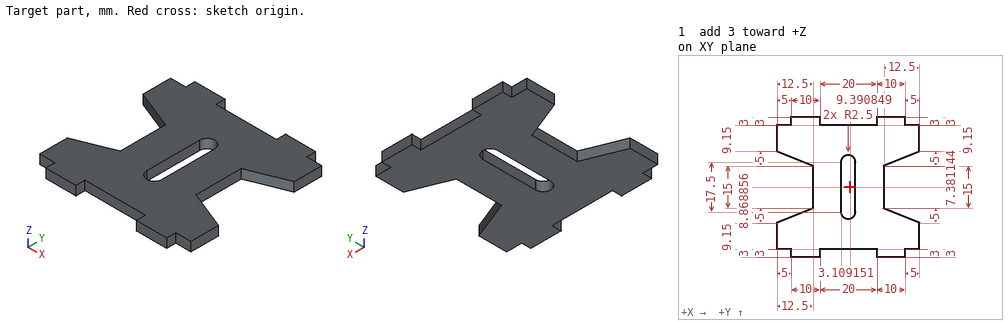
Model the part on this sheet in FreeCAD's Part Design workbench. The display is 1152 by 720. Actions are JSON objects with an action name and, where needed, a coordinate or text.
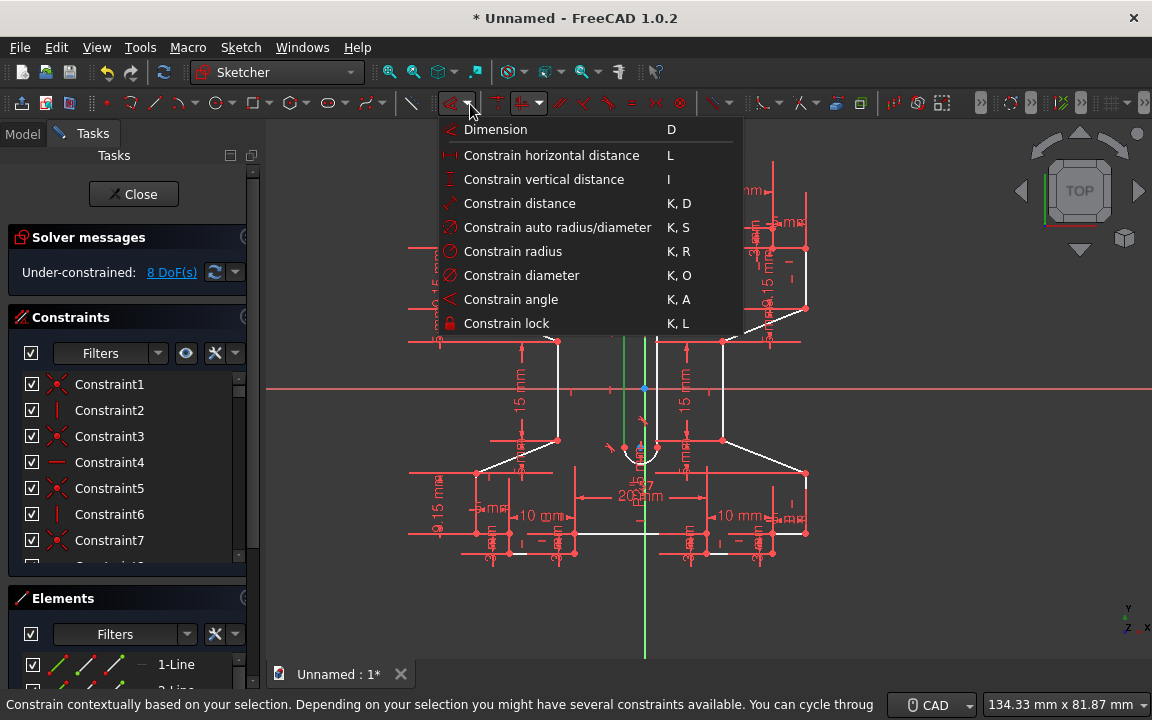
{"action": "left_click", "coordinate": [591, 179]}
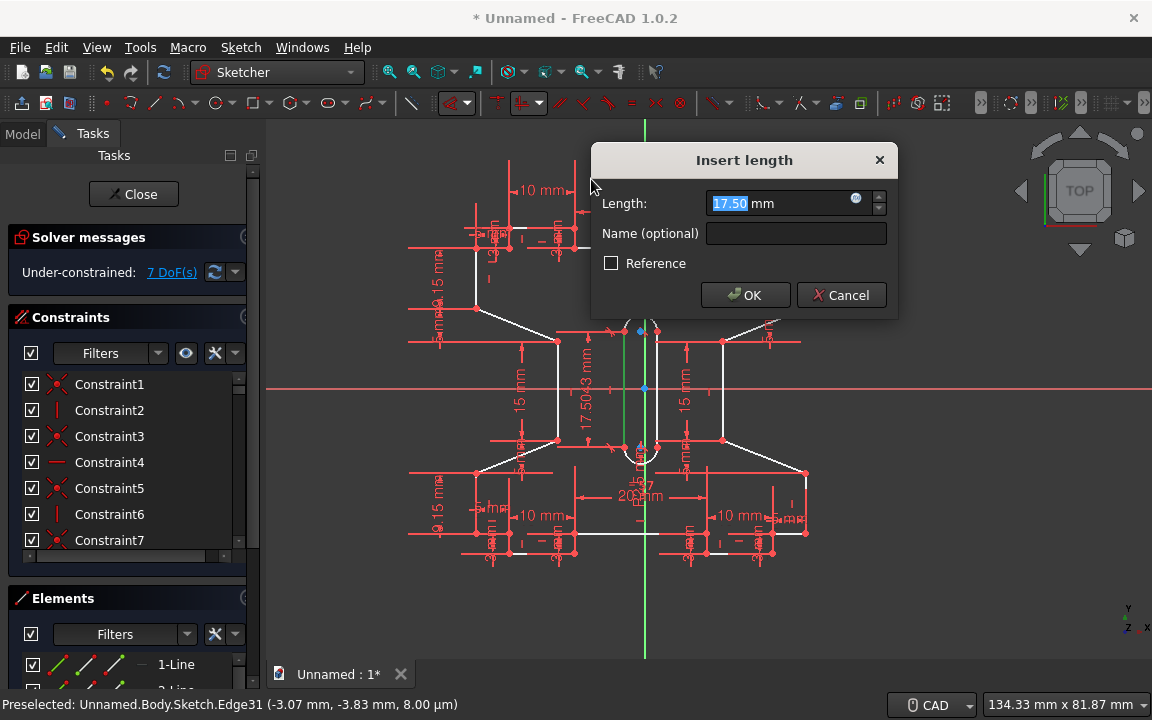
{"action": "type", "text": "17.5"}
{"action": "key", "text": "Return"}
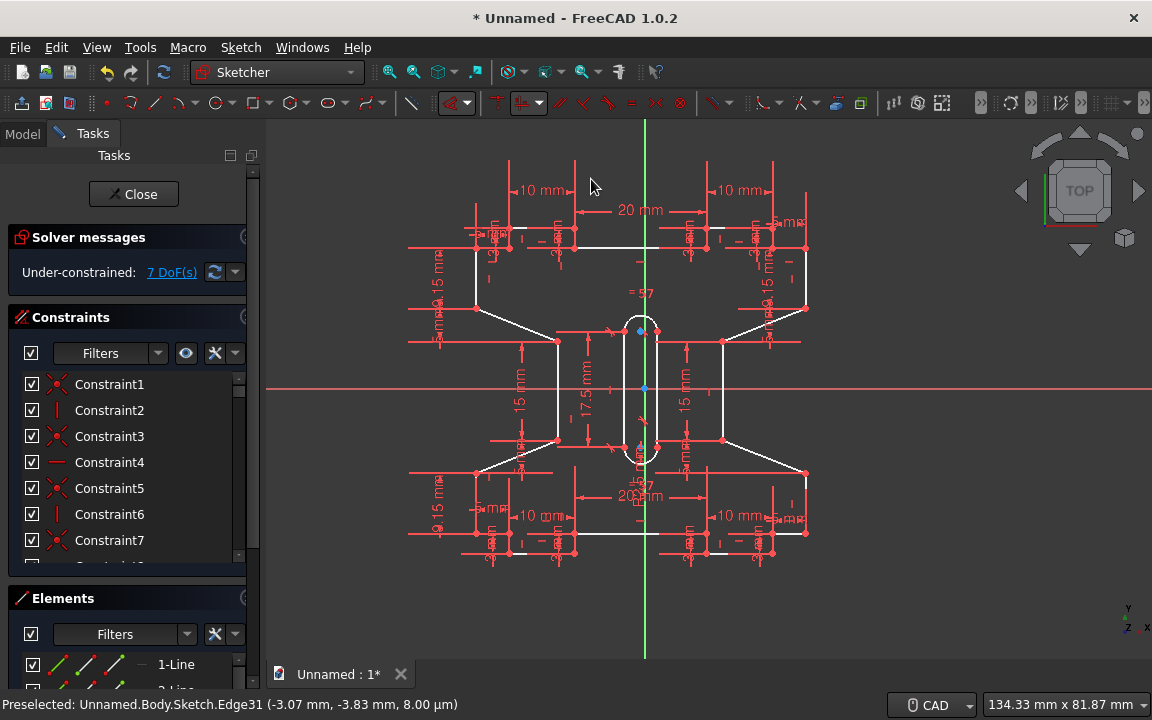
{"action": "left_click", "coordinate": [748, 332]}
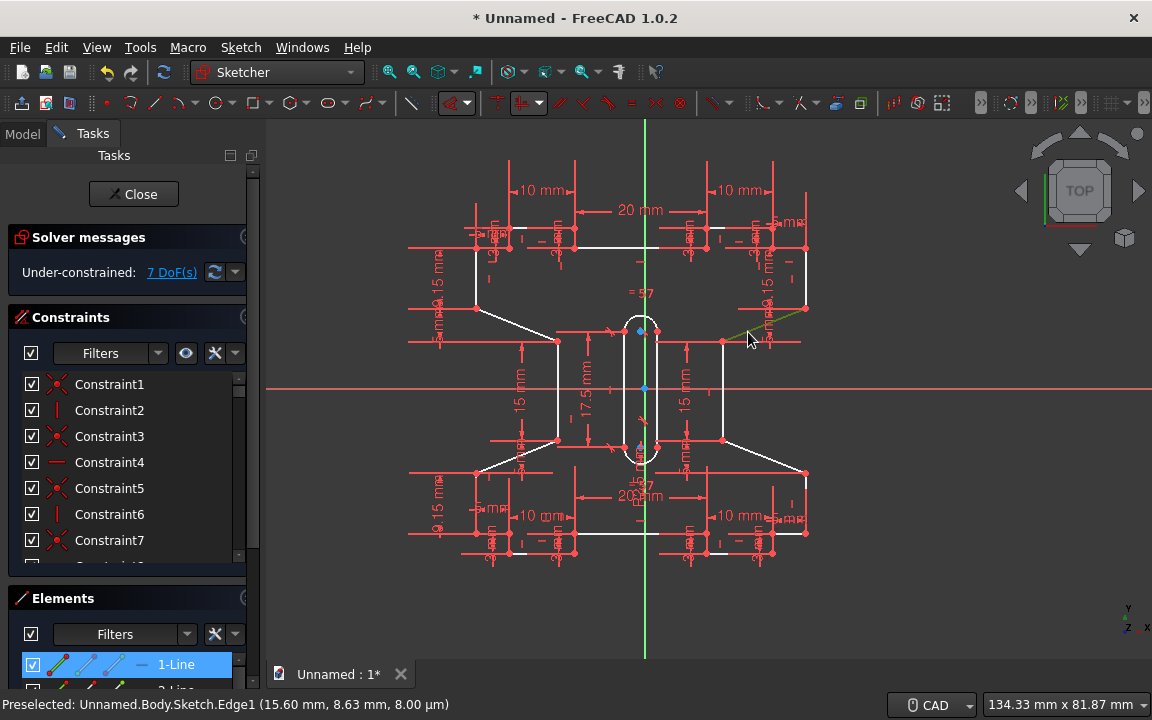
{"action": "left_click", "coordinate": [470, 104]}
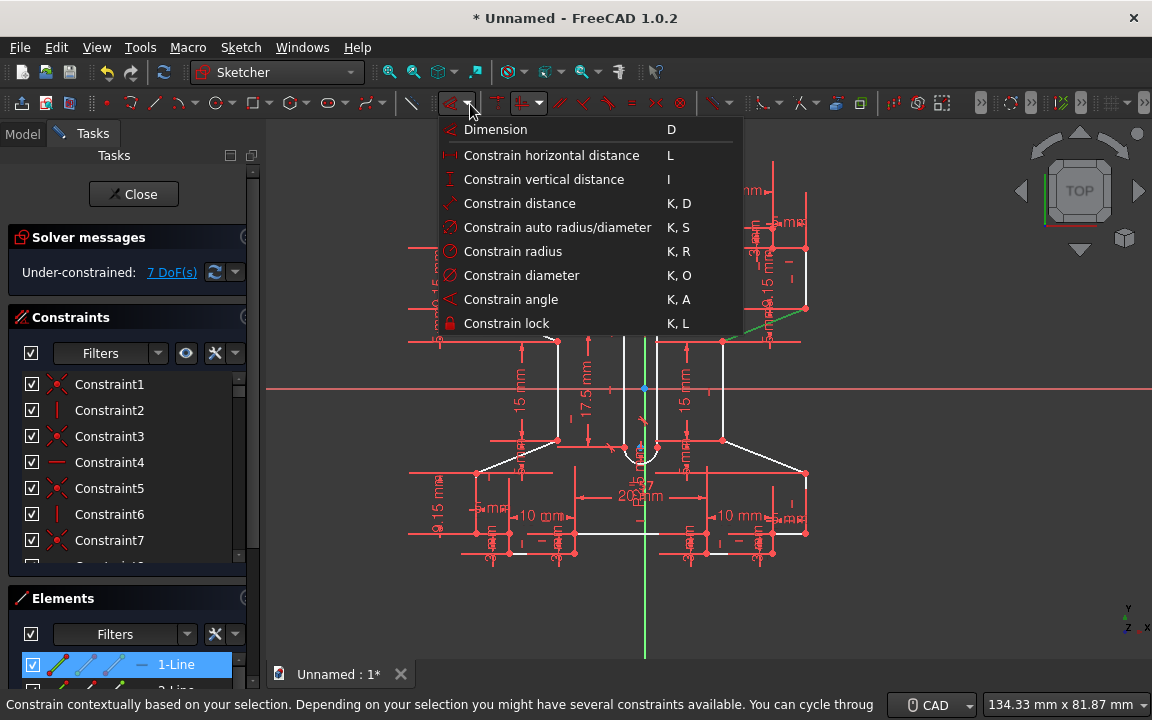
{"action": "left_click", "coordinate": [591, 155]}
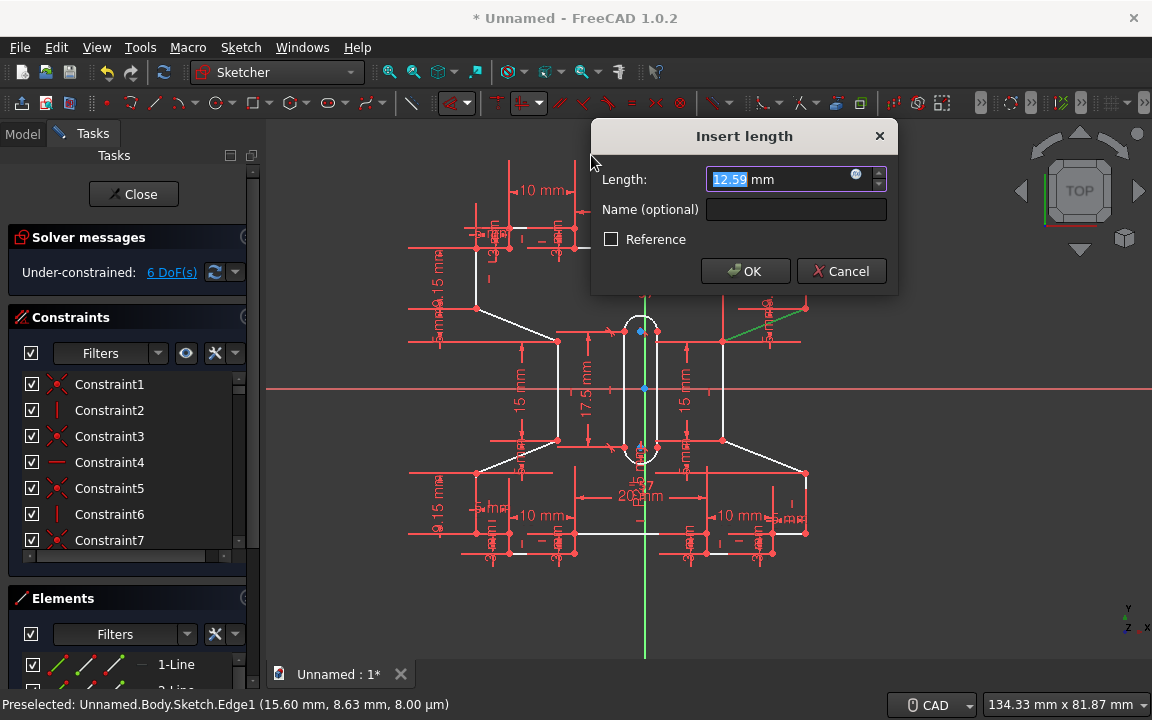
{"action": "type", "text": "12.5"}
{"action": "key", "text": "Return"}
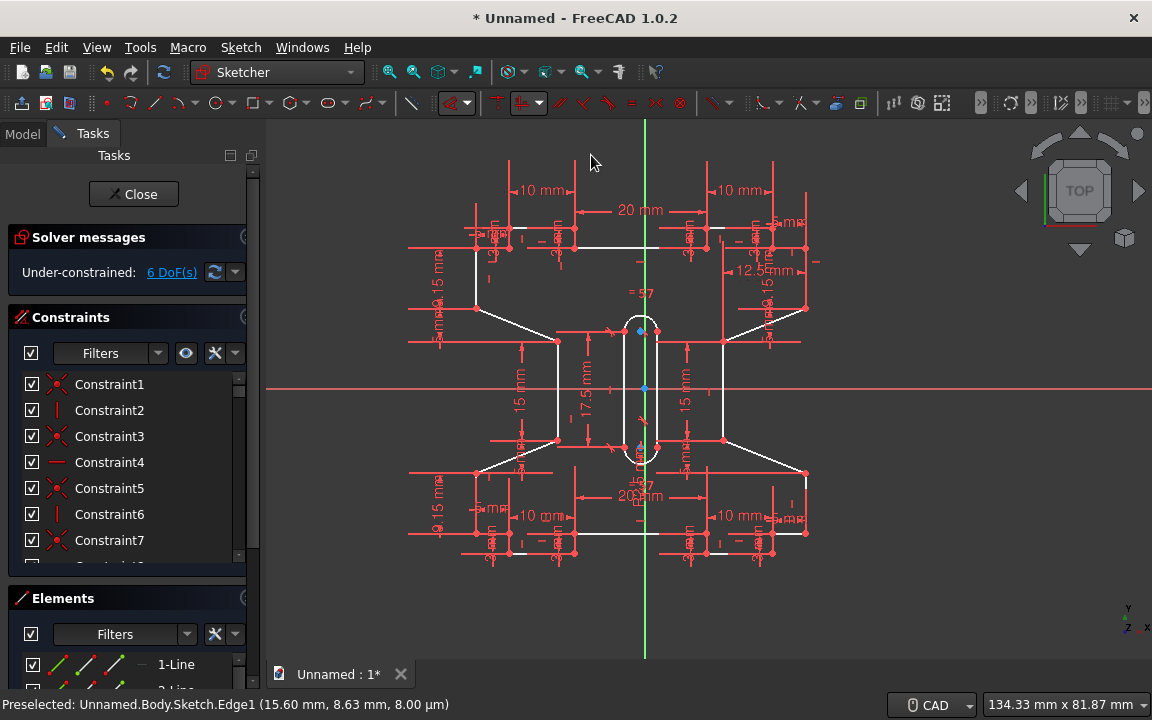
{"action": "left_click", "coordinate": [501, 318]}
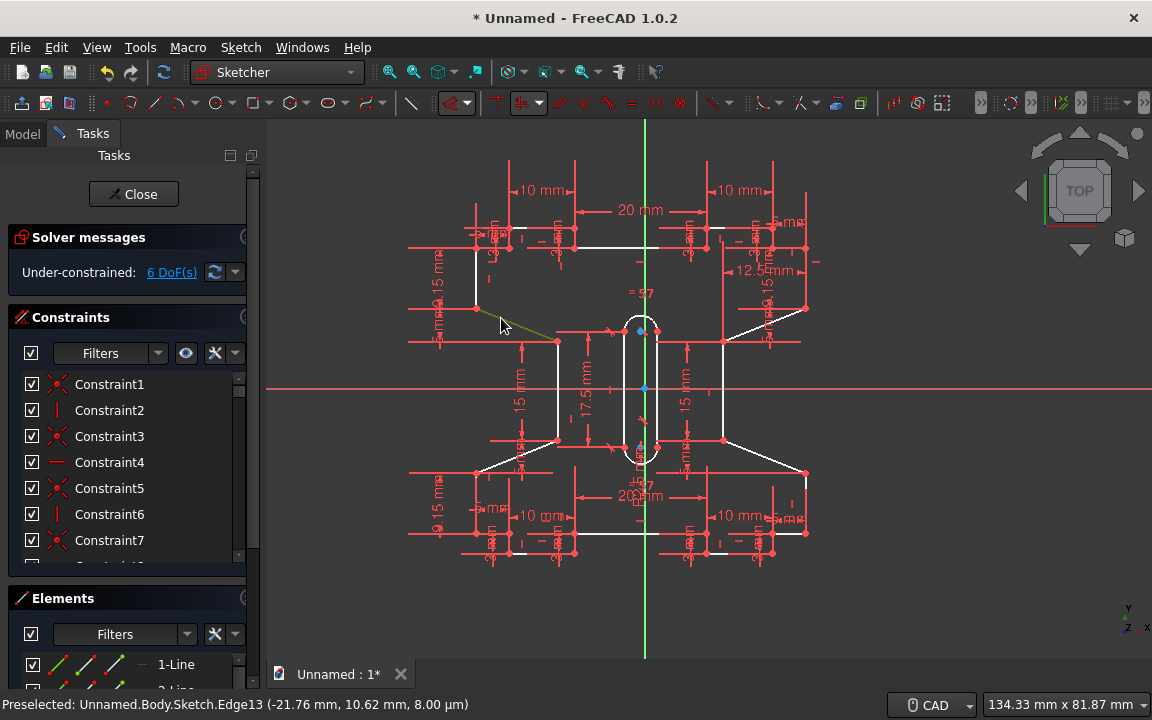
{"action": "left_click", "coordinate": [470, 104]}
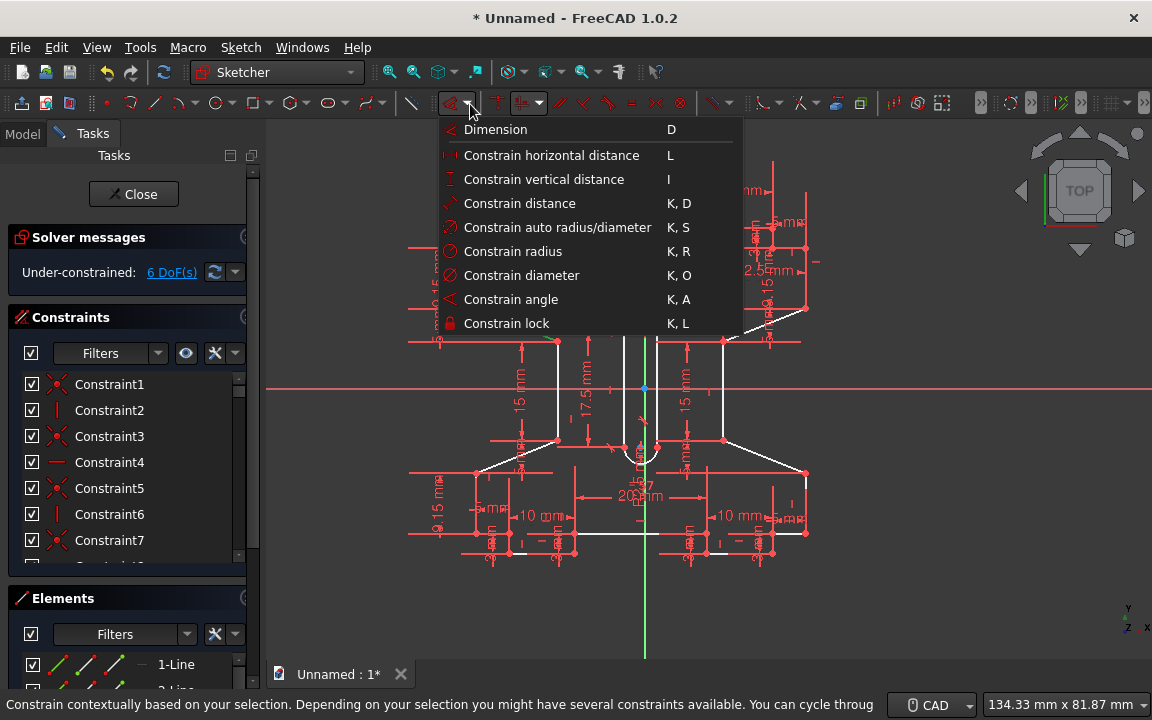
{"action": "left_click", "coordinate": [591, 155]}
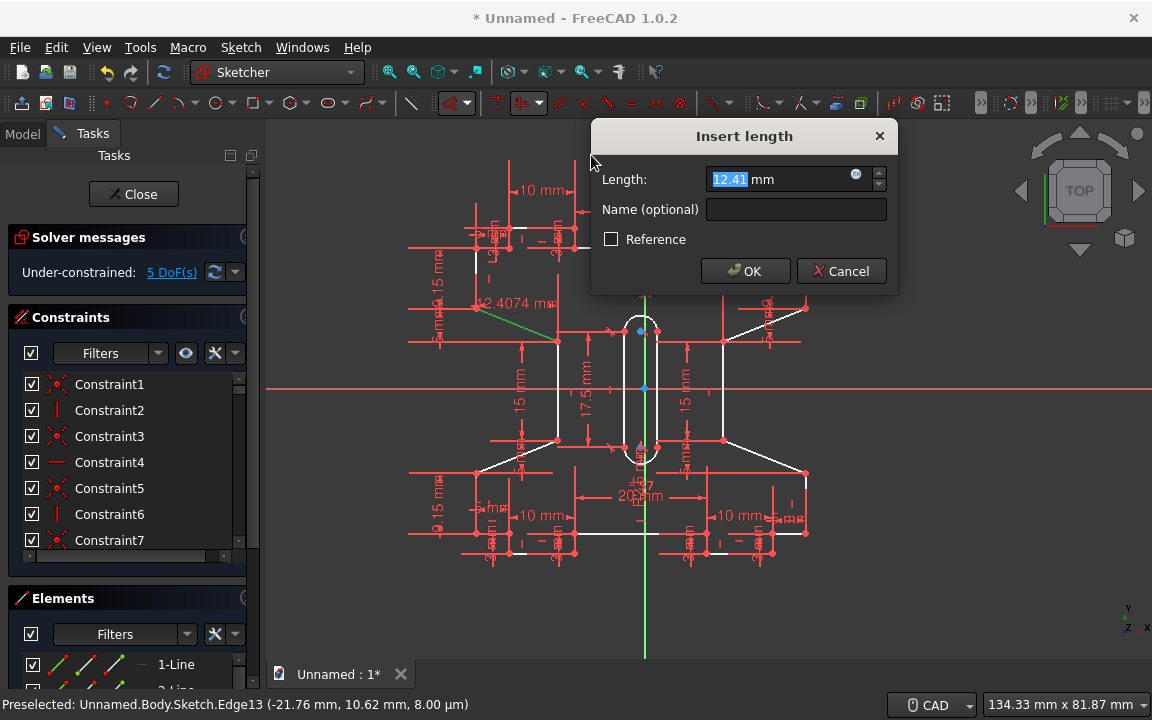
{"action": "type", "text": "12.5"}
{"action": "key", "text": "Return"}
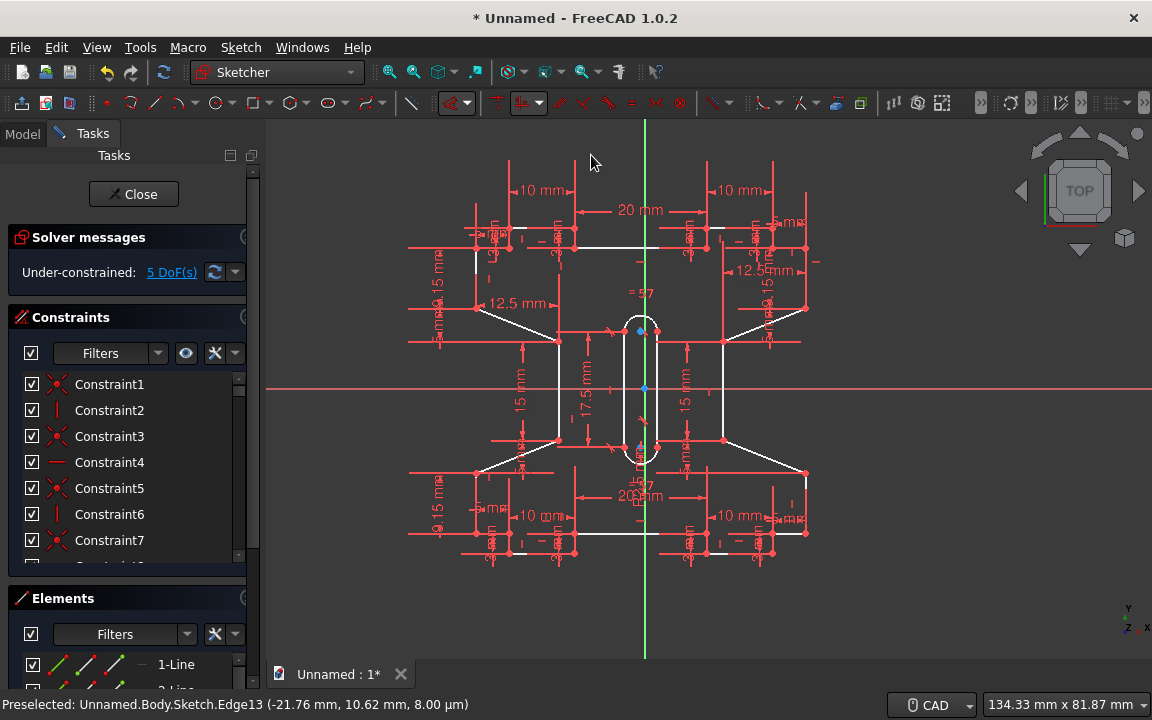
{"action": "left_click", "coordinate": [534, 450]}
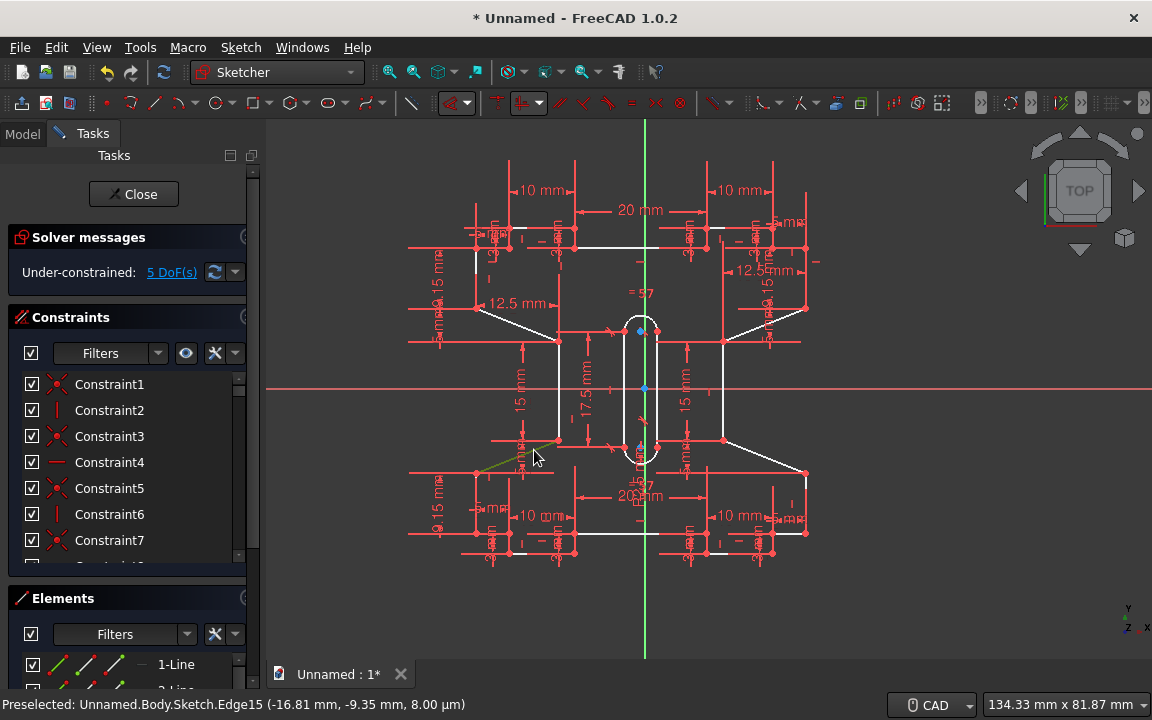
{"action": "key", "text": "l"}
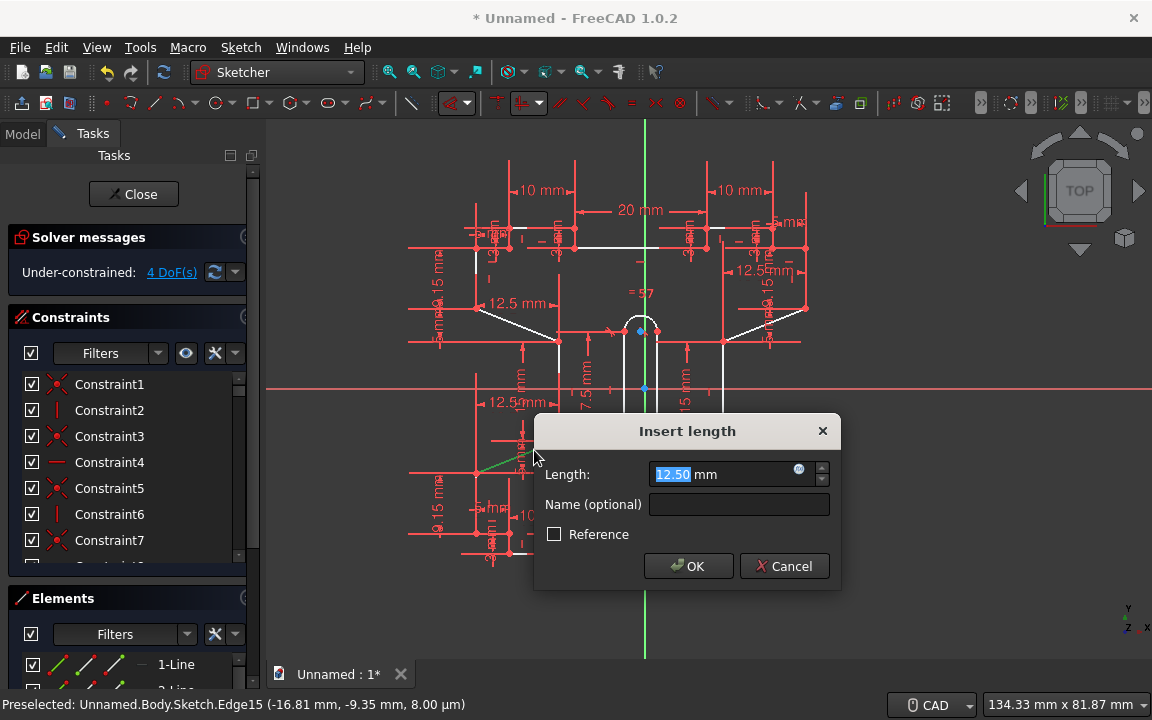
{"action": "type", "text": "12.5"}
{"action": "key", "text": "Return"}